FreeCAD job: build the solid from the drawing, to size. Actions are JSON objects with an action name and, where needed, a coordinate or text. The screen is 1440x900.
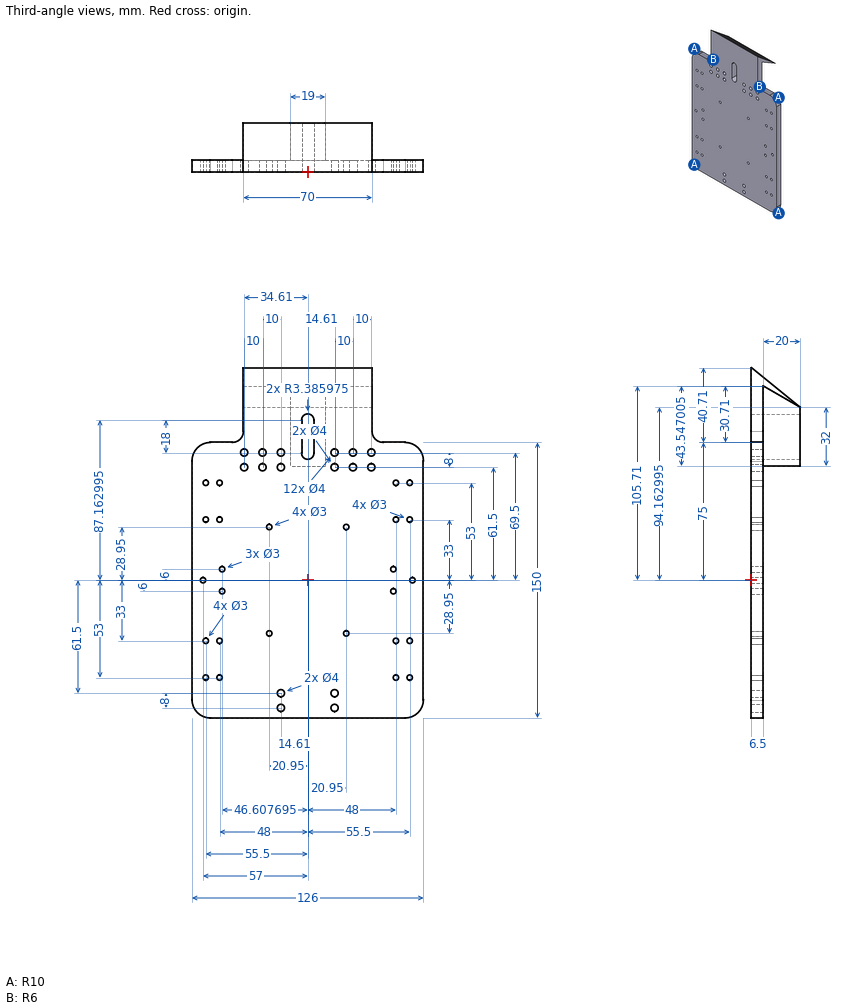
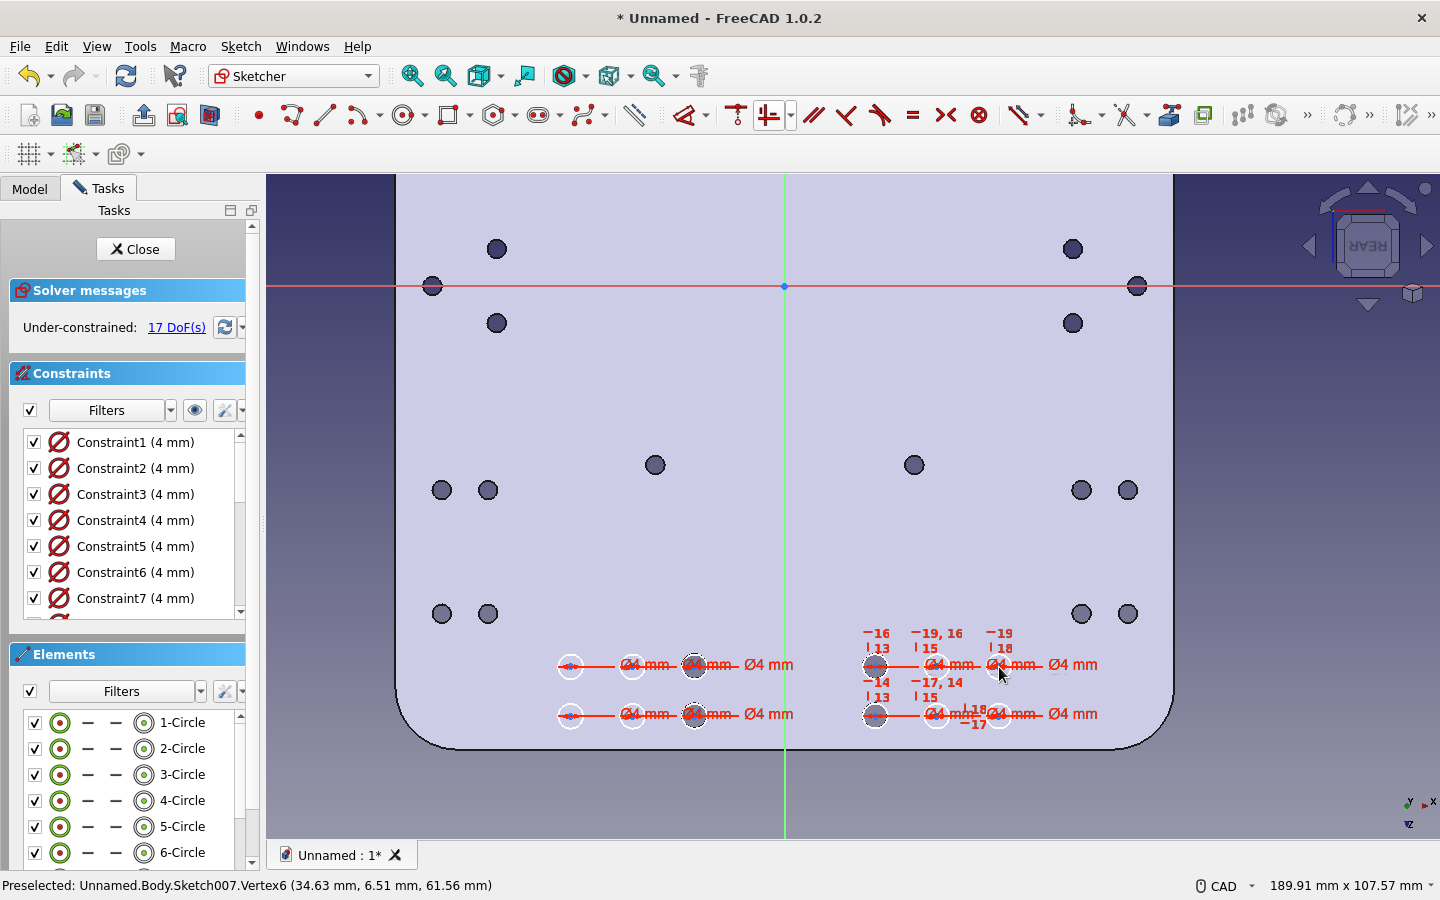
{"action": "left_click", "coordinate": [875, 667]}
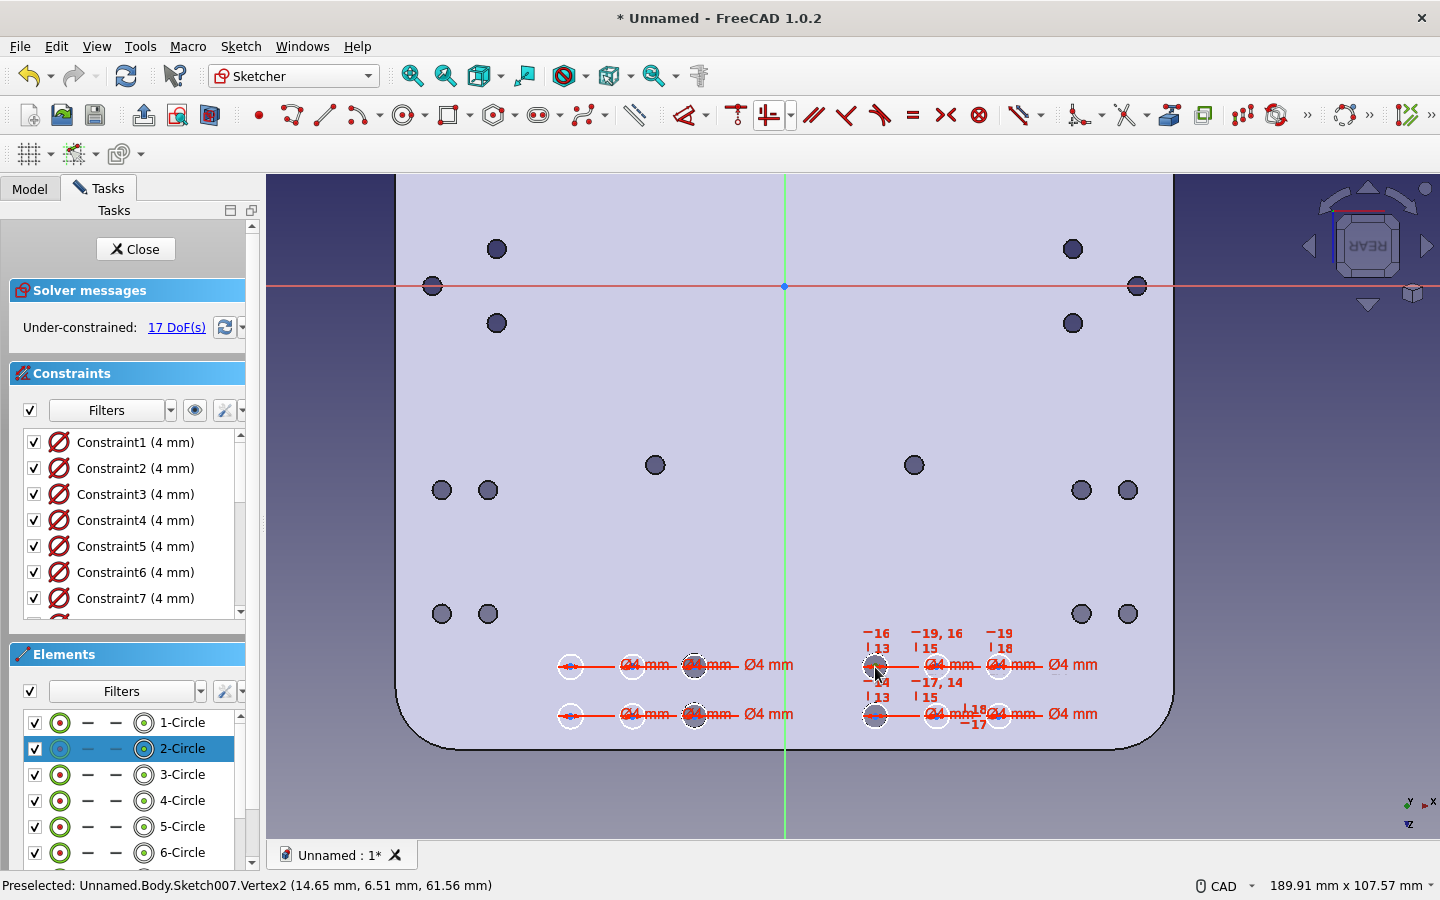
{"action": "left_click", "coordinate": [571, 667]}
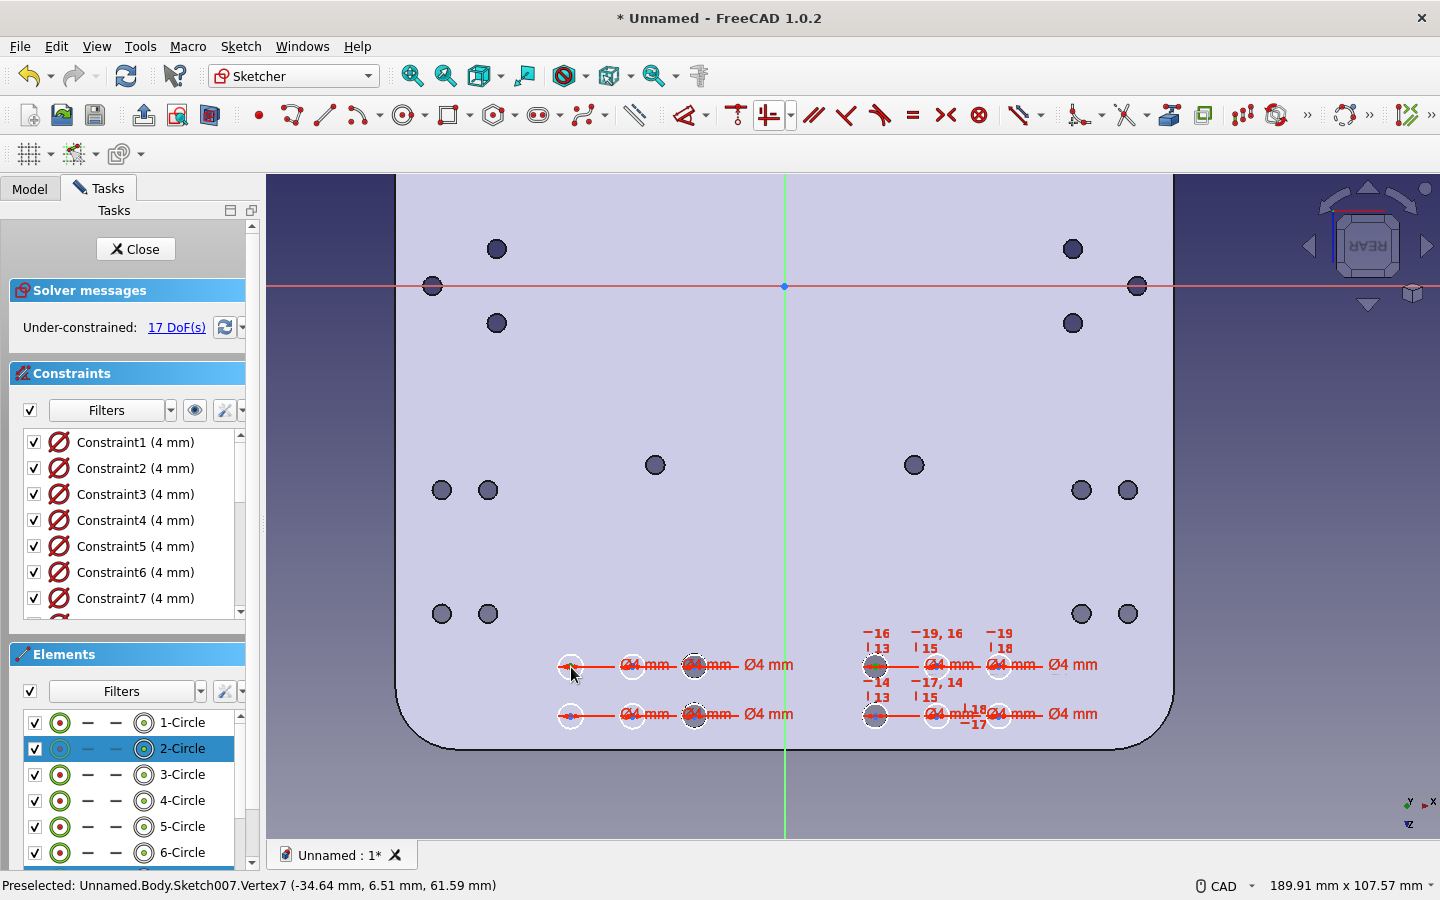
{"action": "key", "text": "h"}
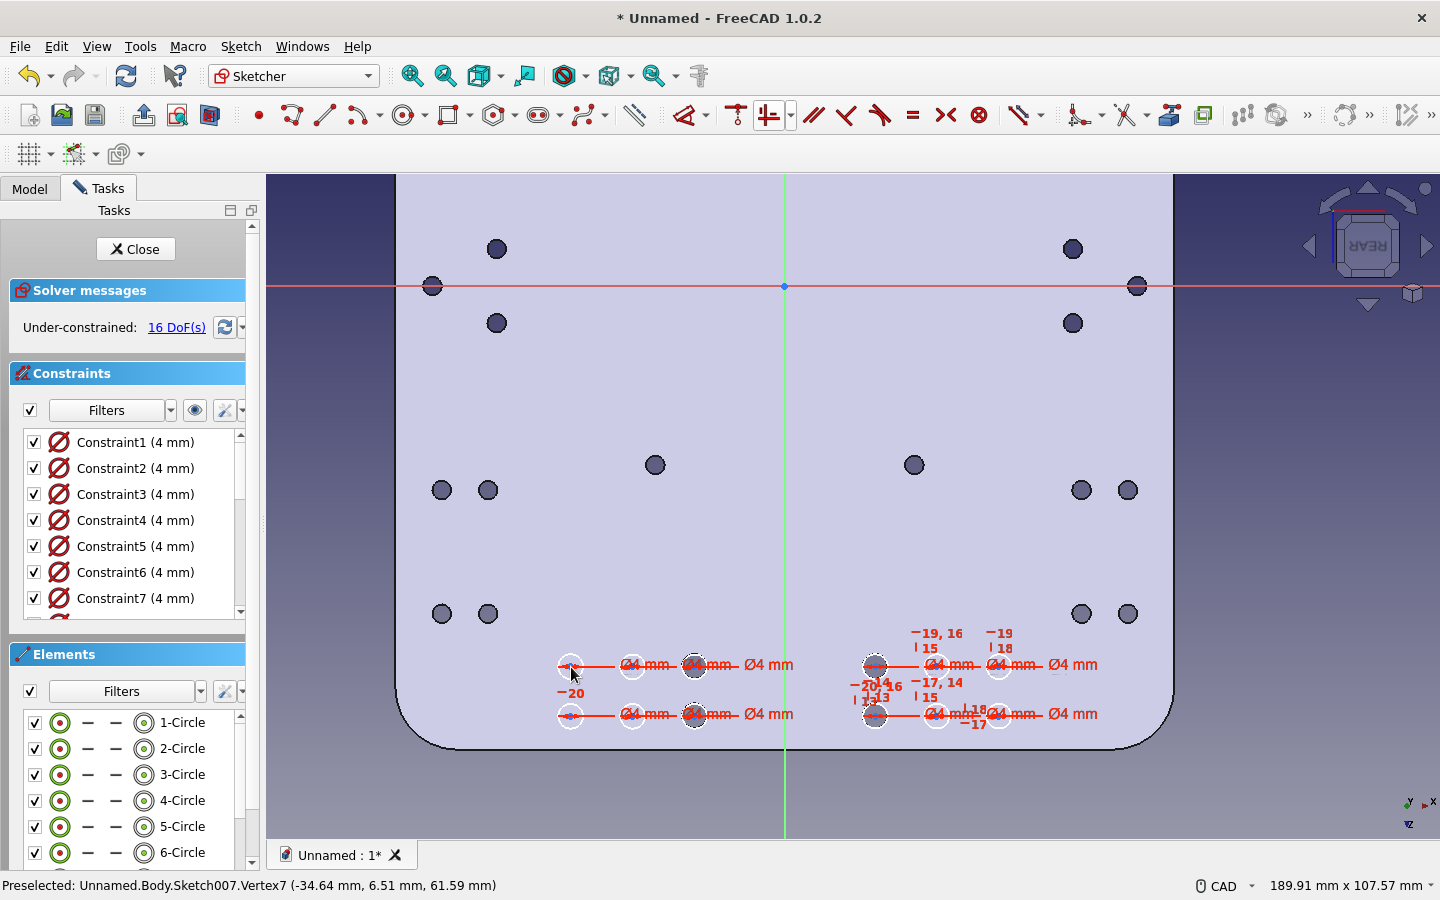
{"action": "left_click", "coordinate": [571, 667]}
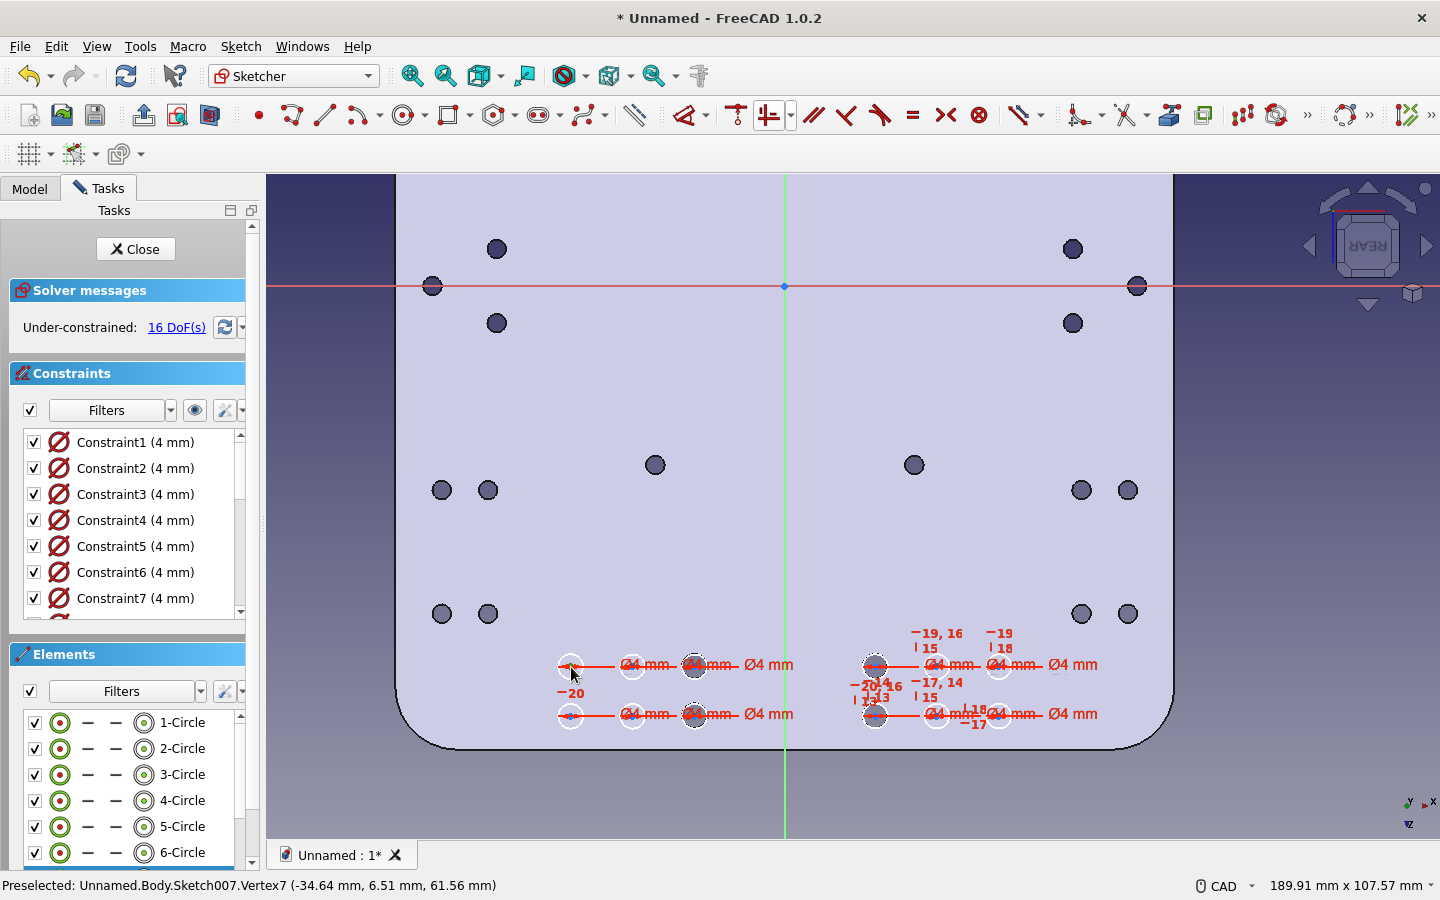
{"action": "left_click", "coordinate": [571, 716]}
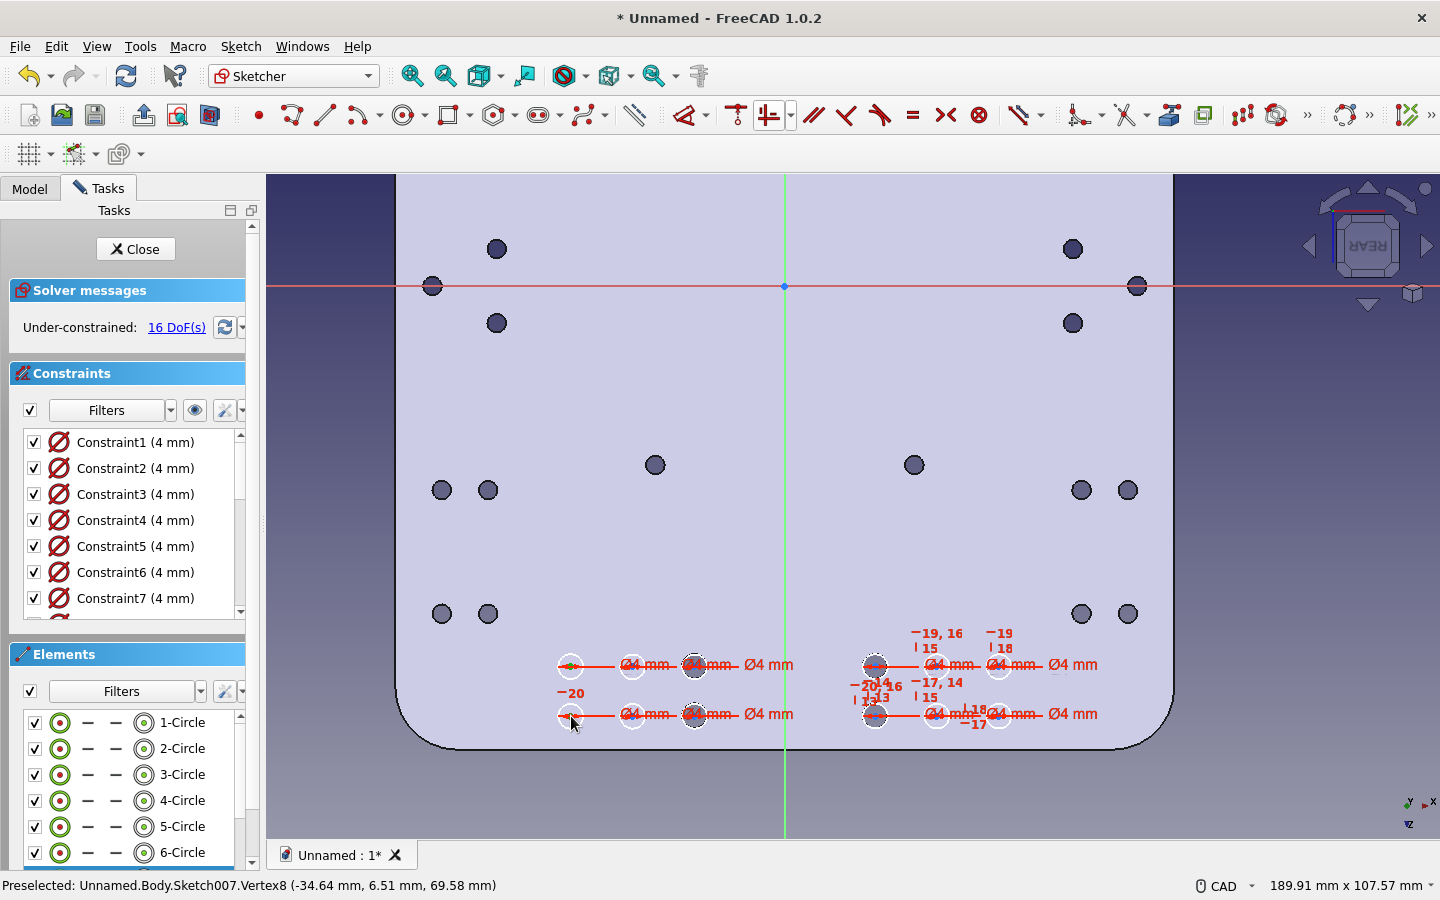
{"action": "key", "text": "v"}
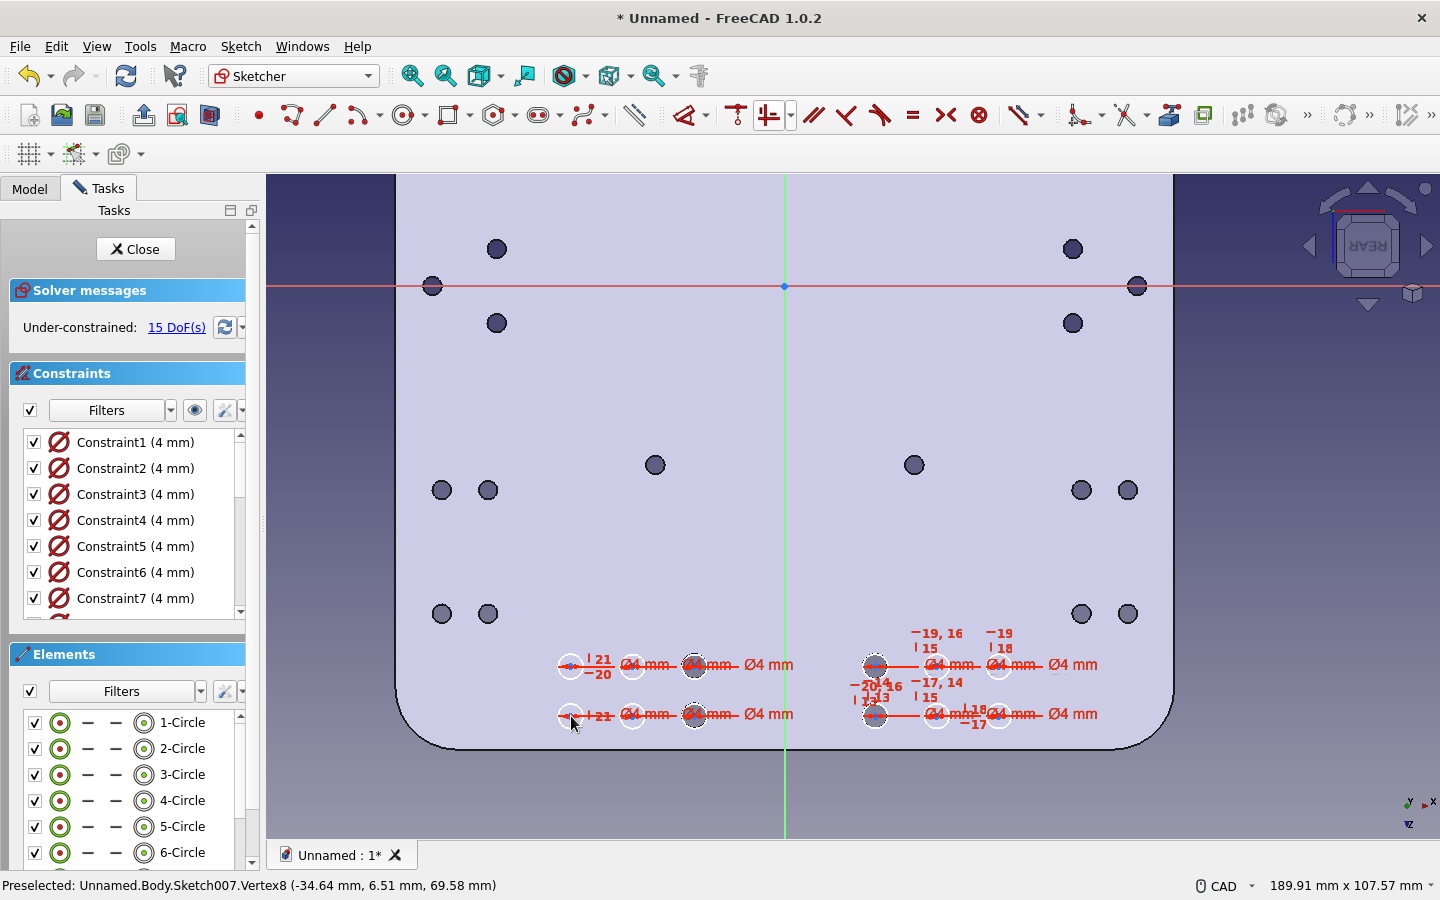
{"action": "left_click", "coordinate": [875, 716]}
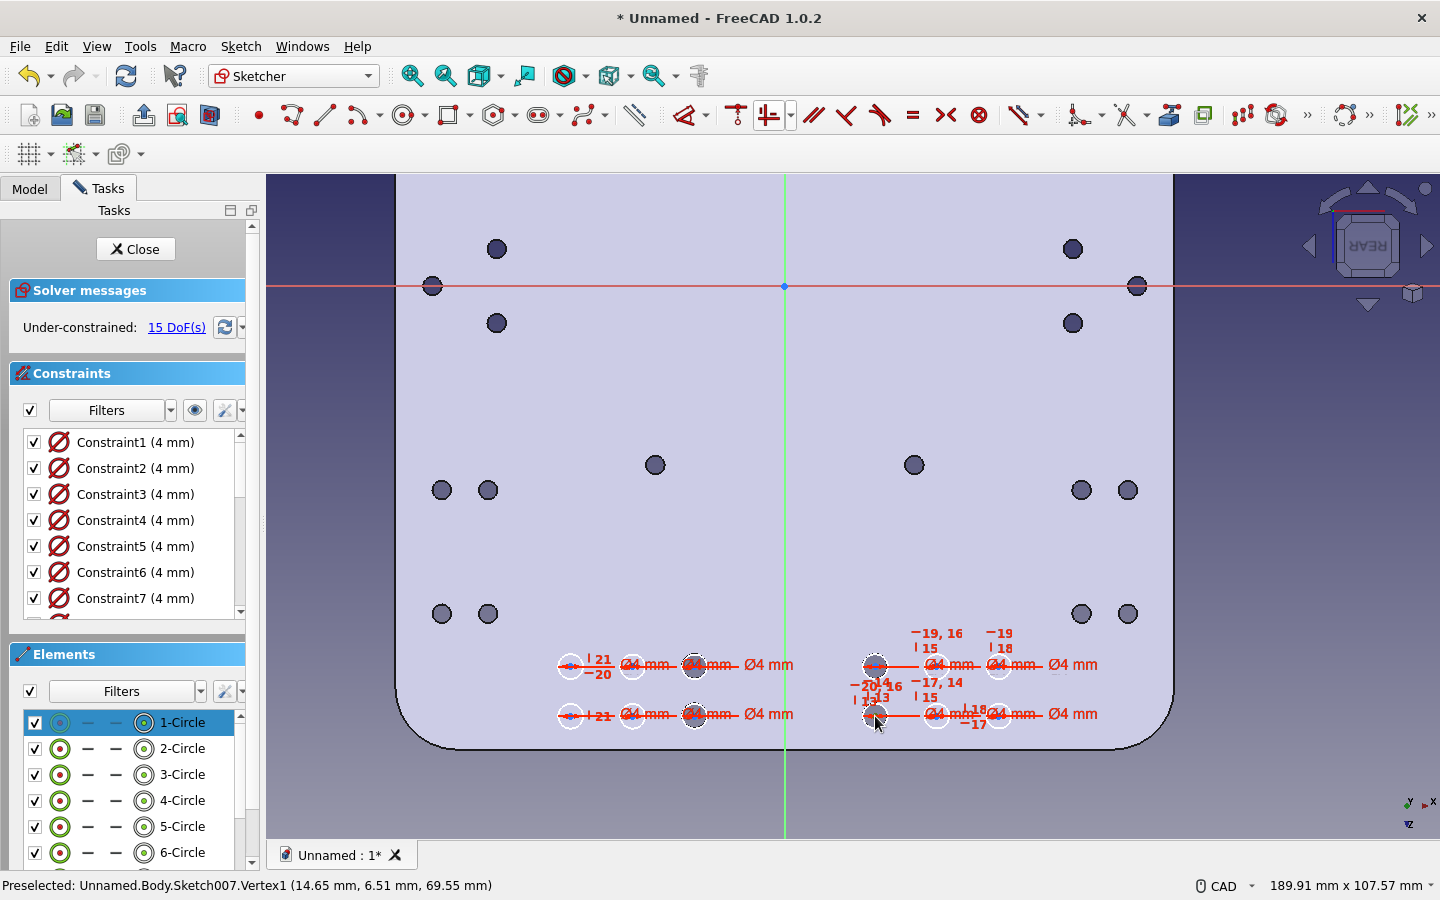
{"action": "left_click", "coordinate": [571, 716]}